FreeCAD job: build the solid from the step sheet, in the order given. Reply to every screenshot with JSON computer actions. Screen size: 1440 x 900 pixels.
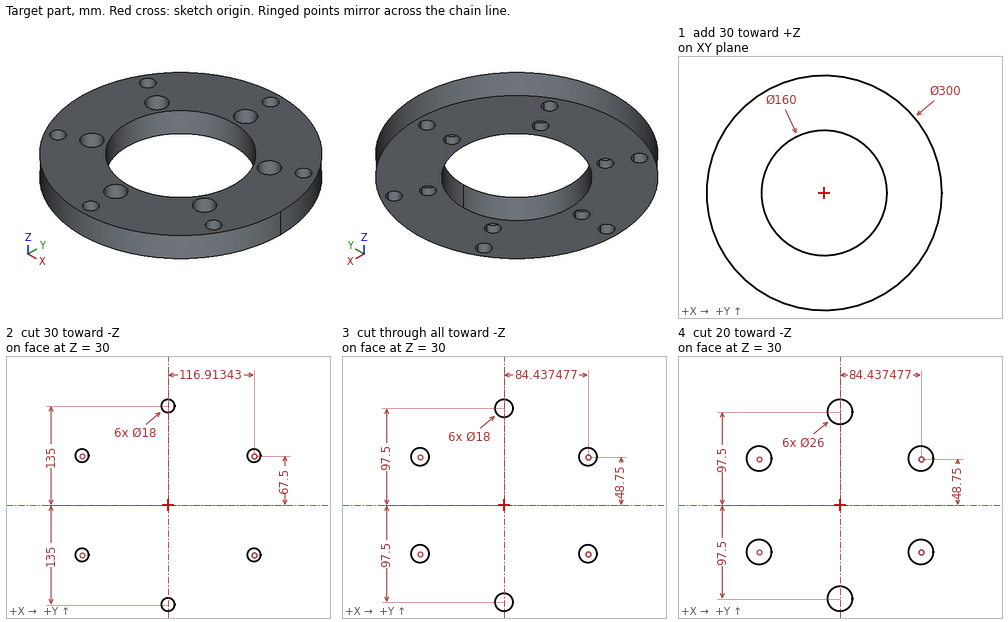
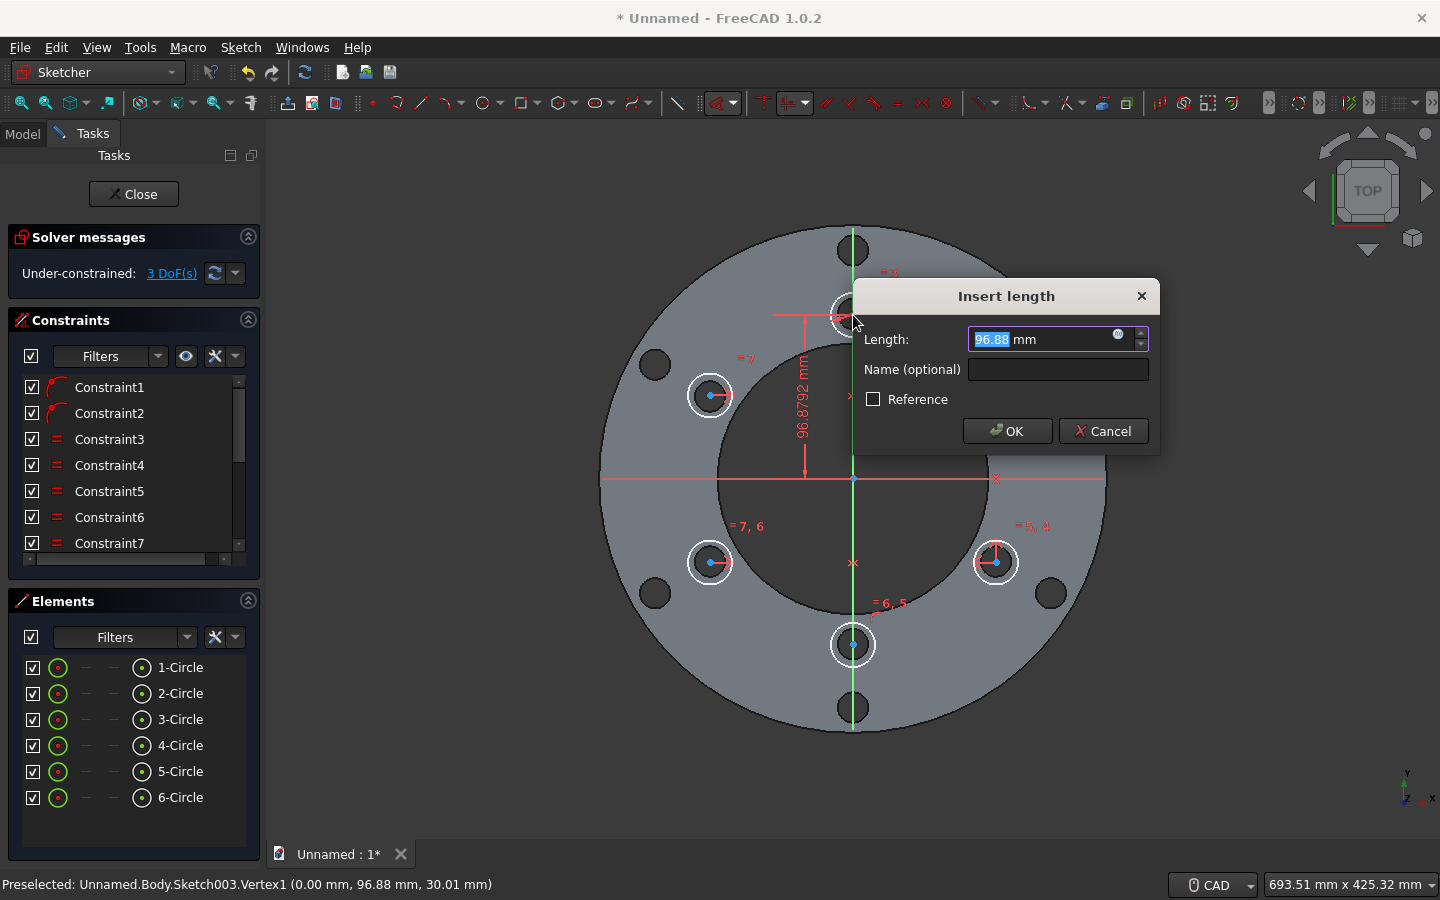
{"action": "type", "text": "97.5"}
{"action": "key", "text": "Return"}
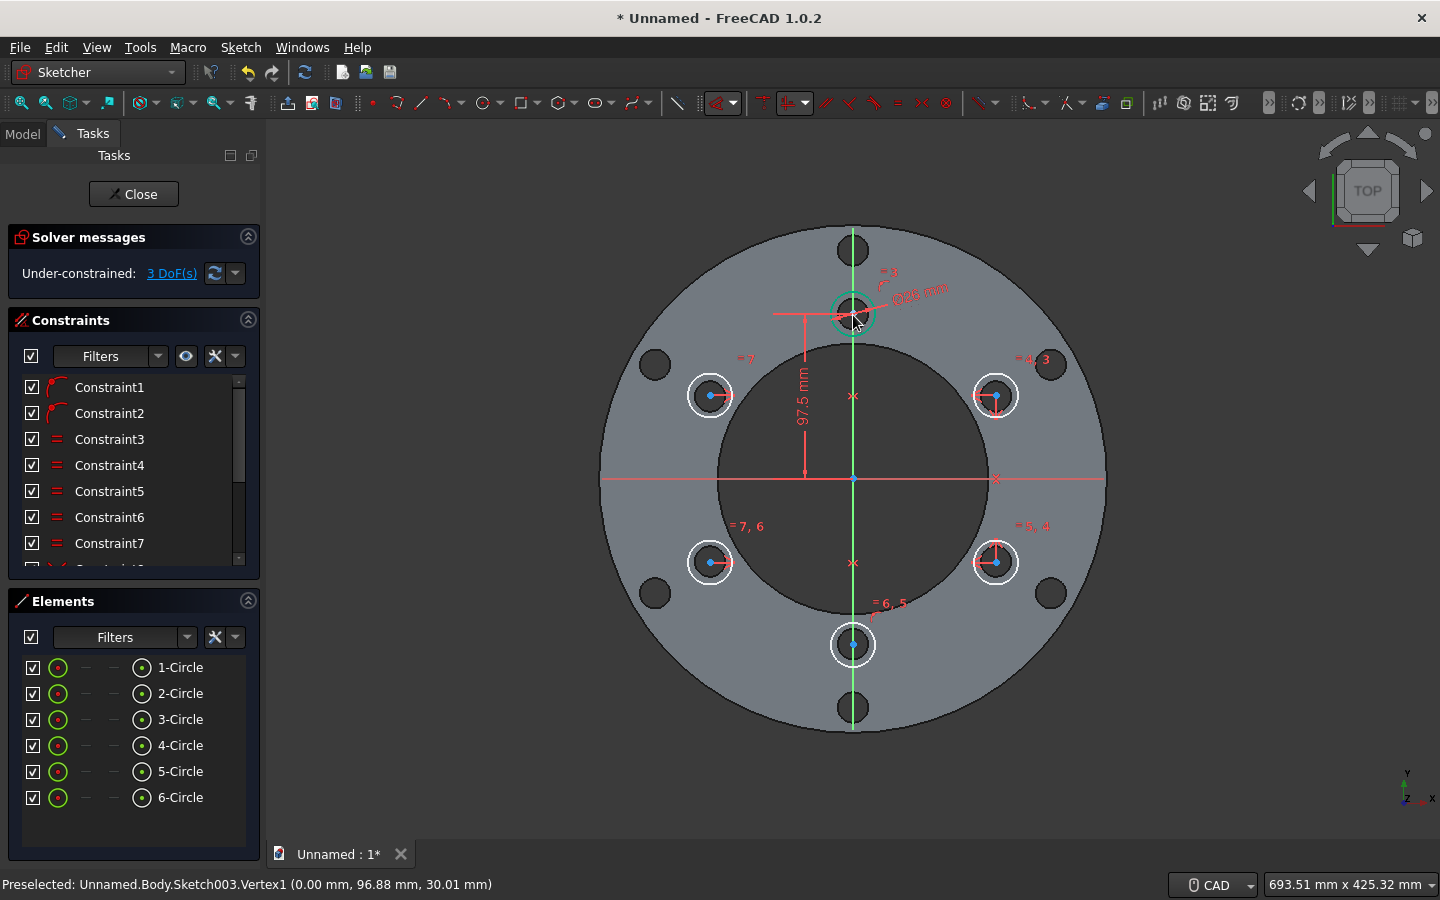
{"action": "left_click", "coordinate": [853, 645]}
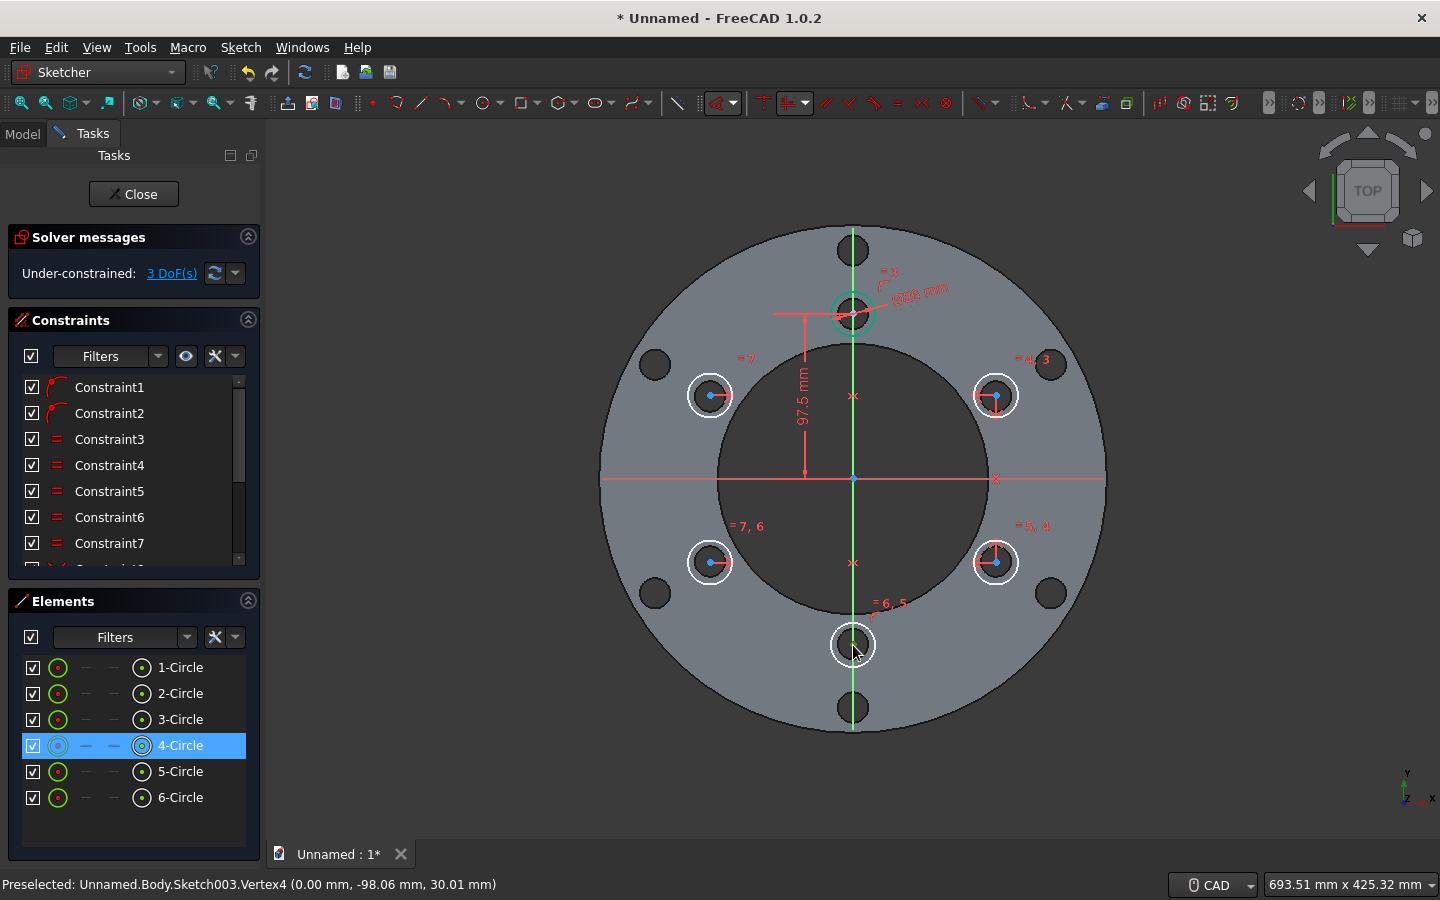
{"action": "key", "text": "i"}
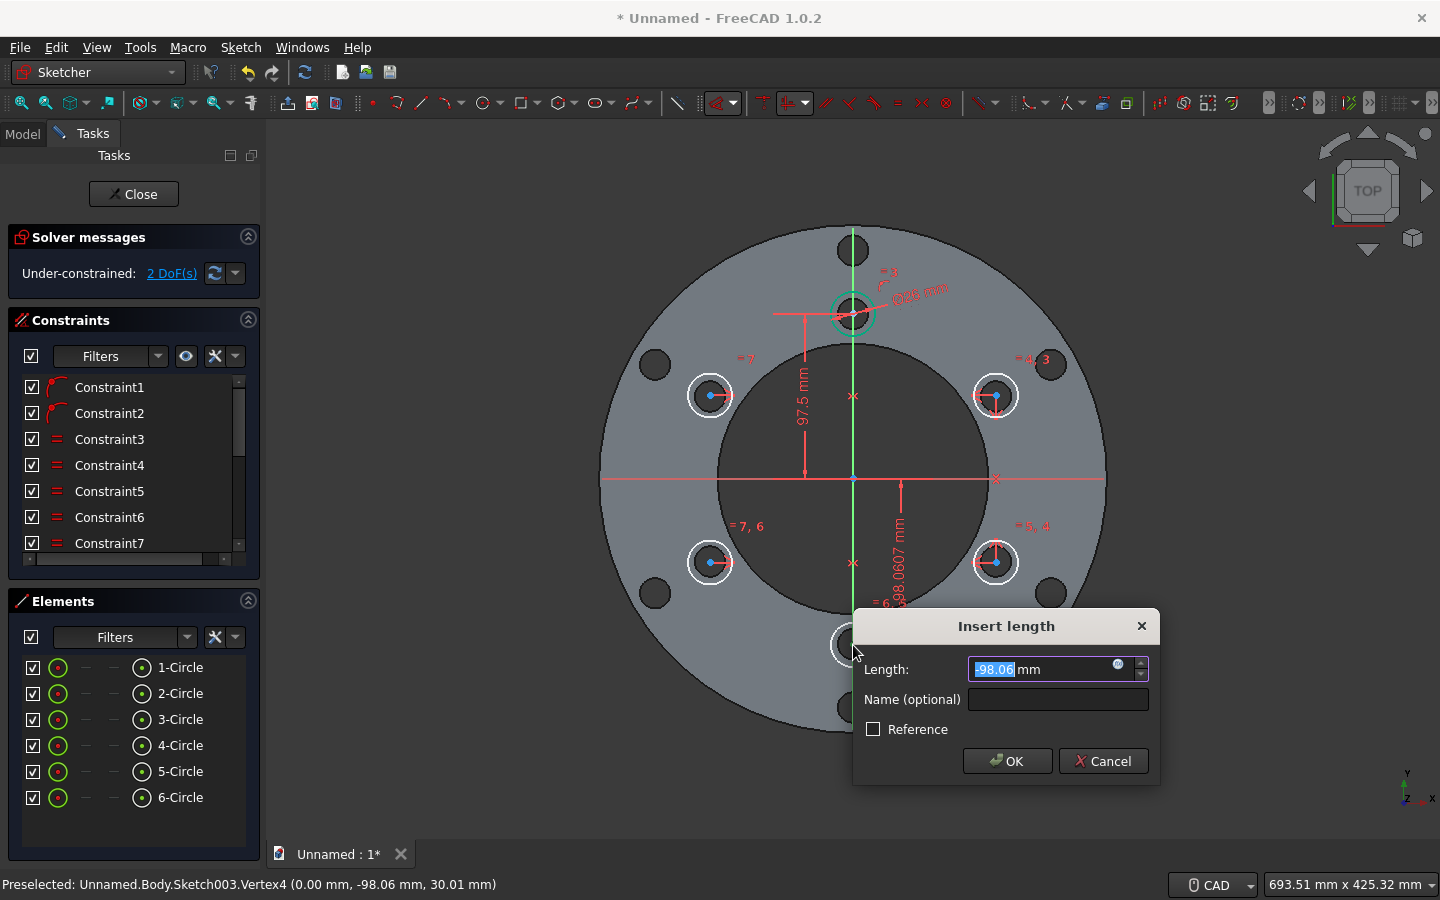
{"action": "type", "text": "-97.5"}
{"action": "key", "text": "Return"}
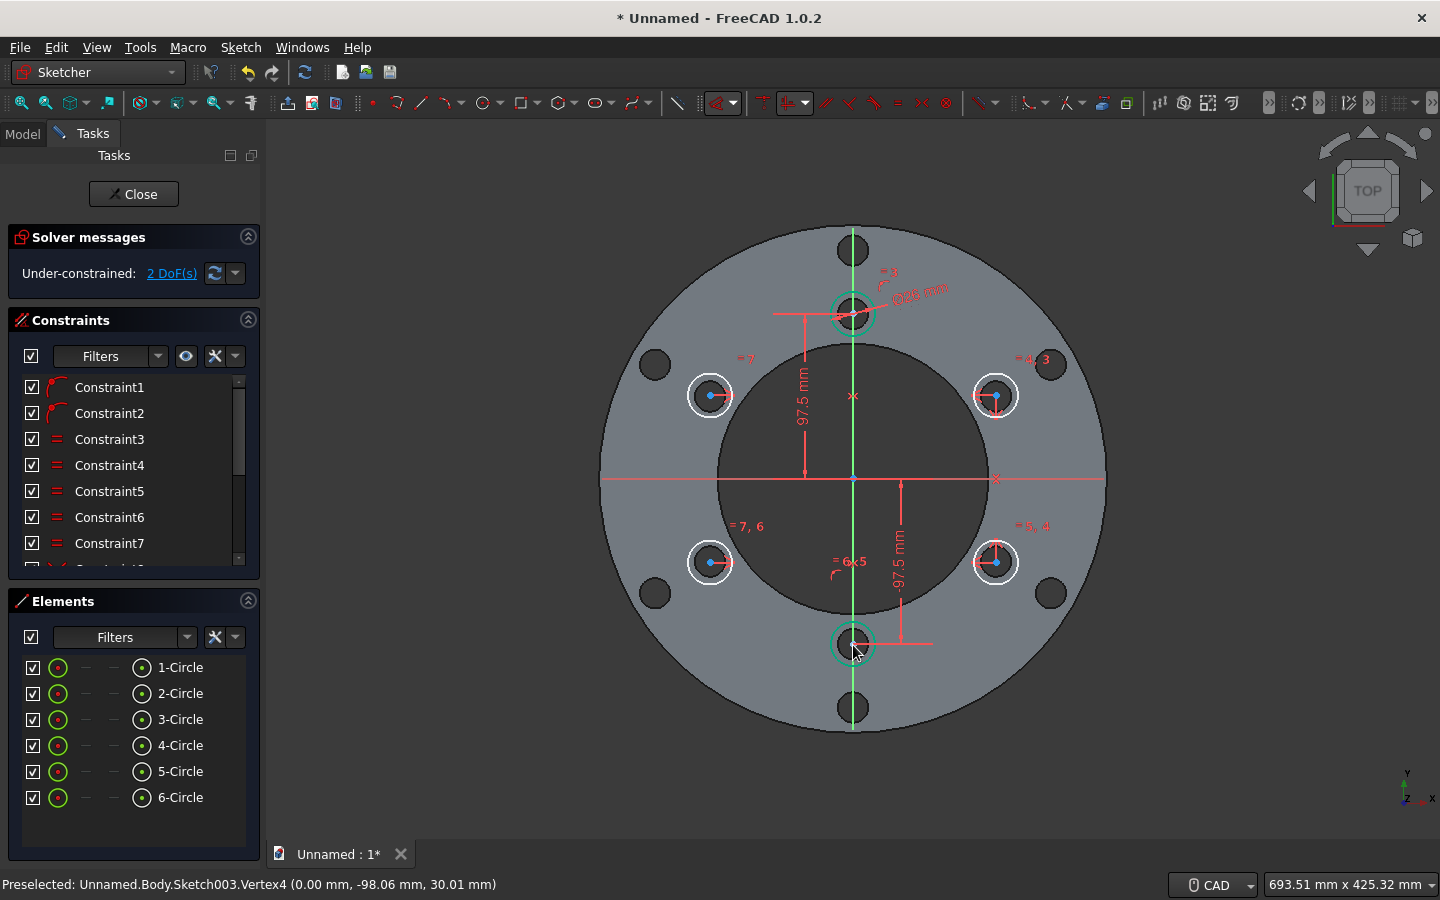
{"action": "left_click", "coordinate": [996, 395]}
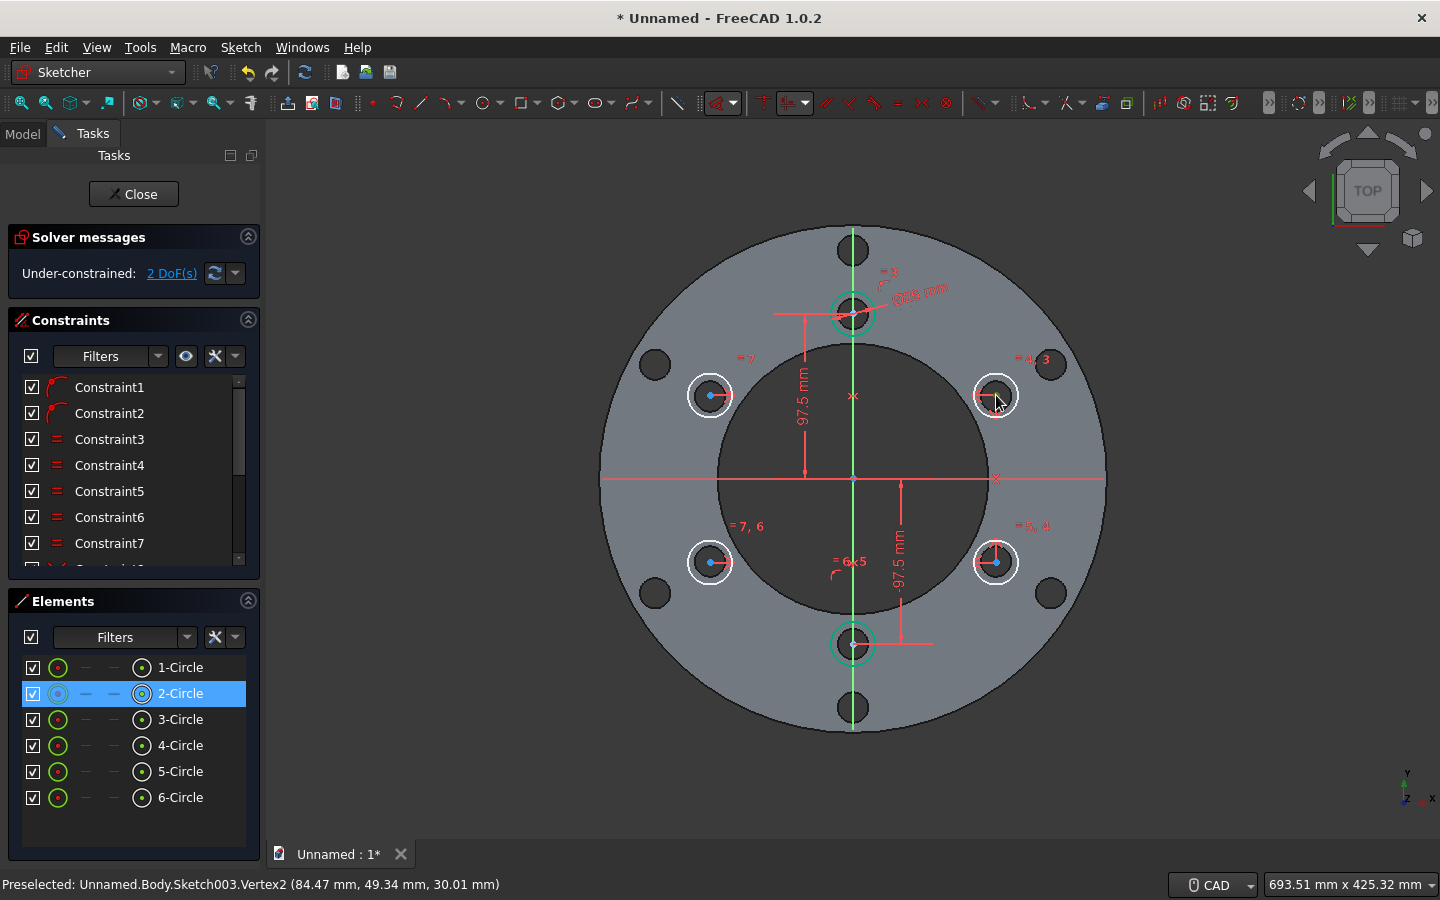
{"action": "key", "text": "i"}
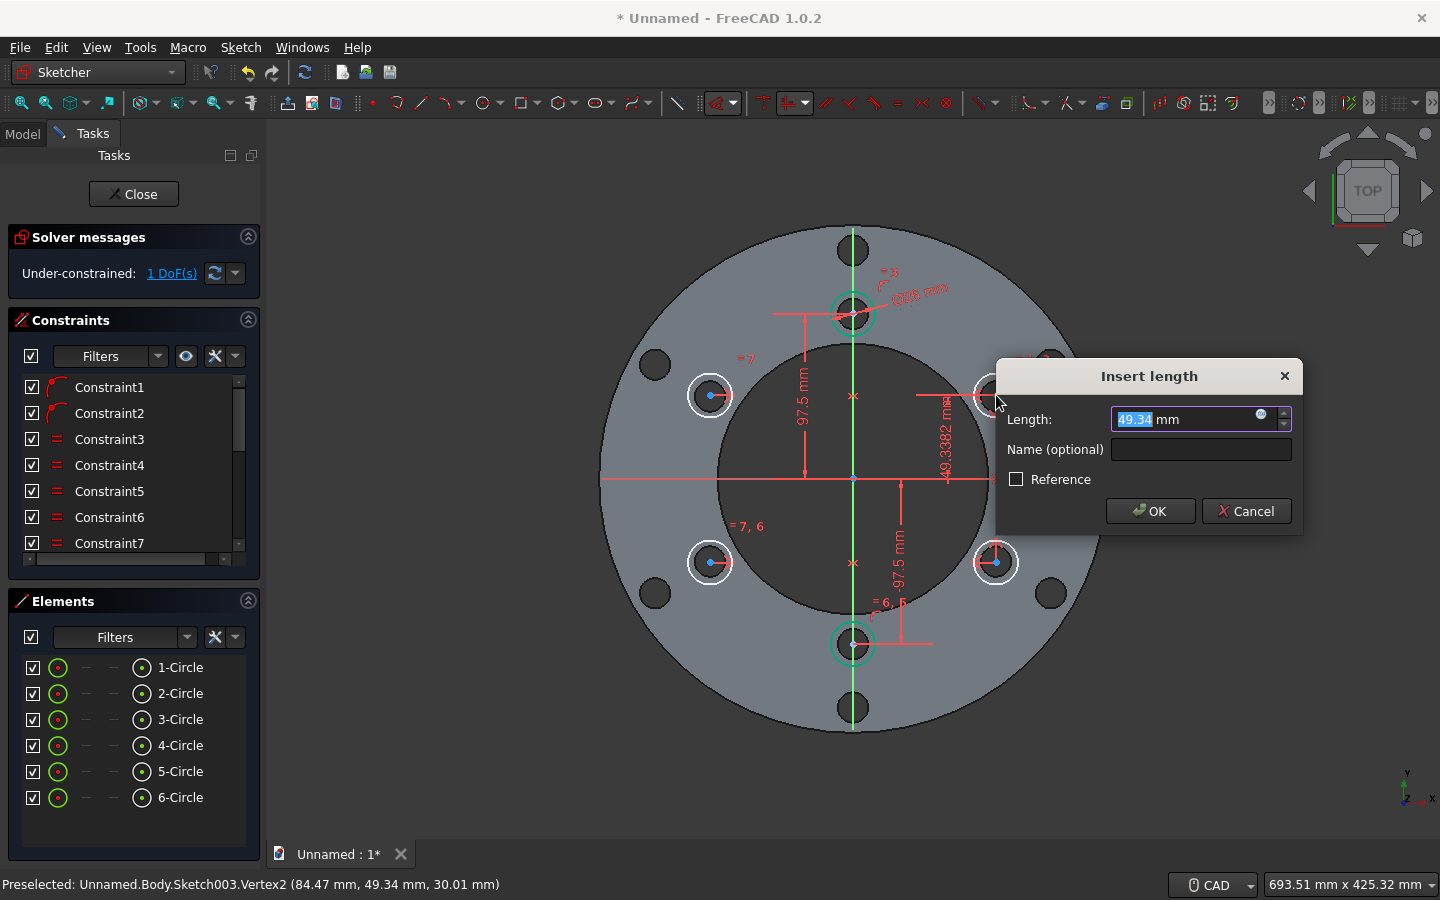
{"action": "type", "text": "48.75"}
{"action": "key", "text": "Return"}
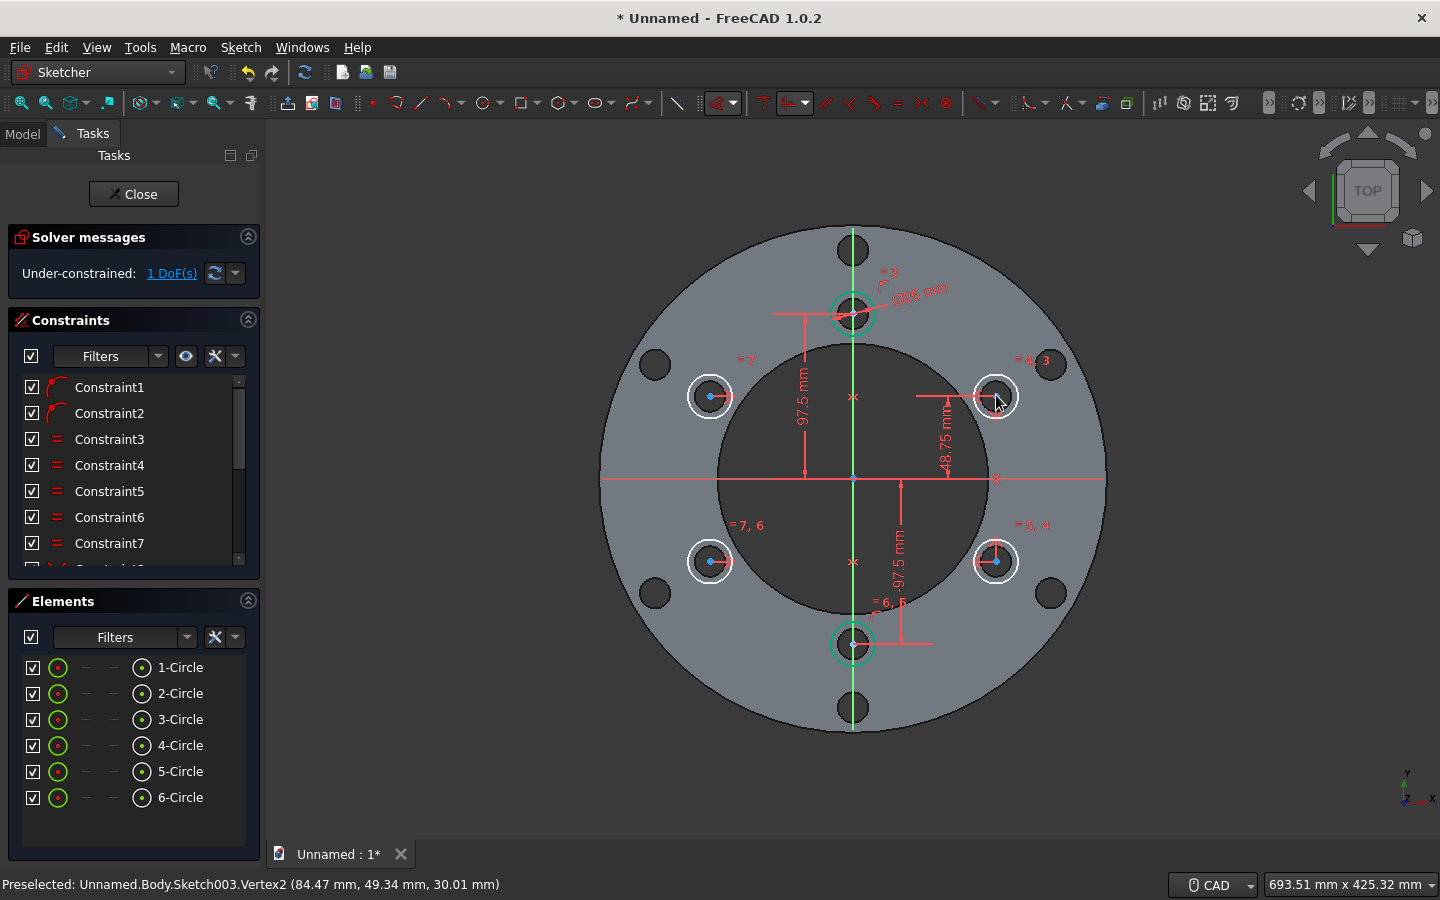
{"action": "left_click", "coordinate": [996, 396]}